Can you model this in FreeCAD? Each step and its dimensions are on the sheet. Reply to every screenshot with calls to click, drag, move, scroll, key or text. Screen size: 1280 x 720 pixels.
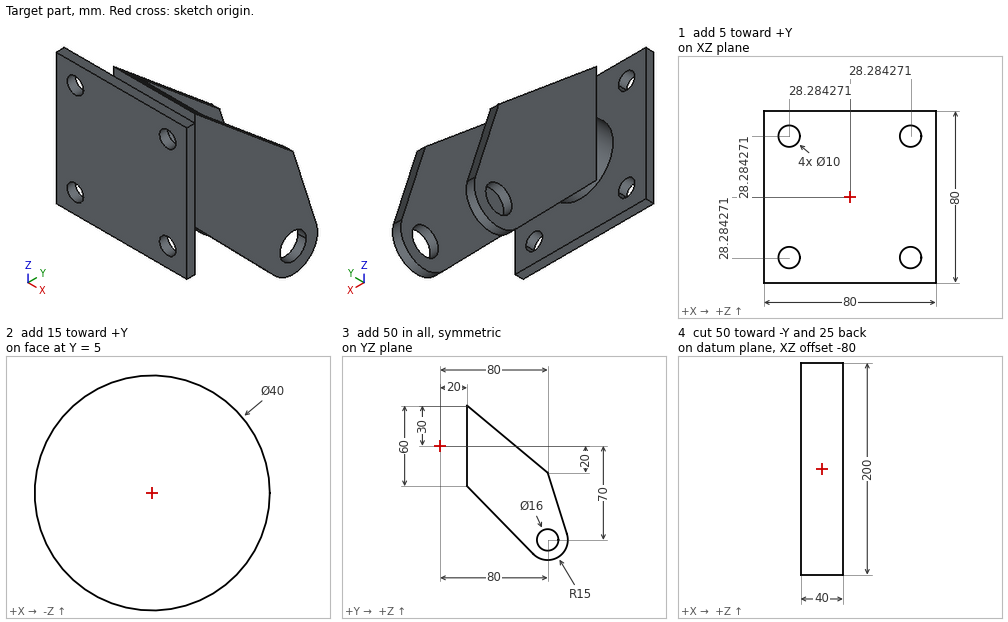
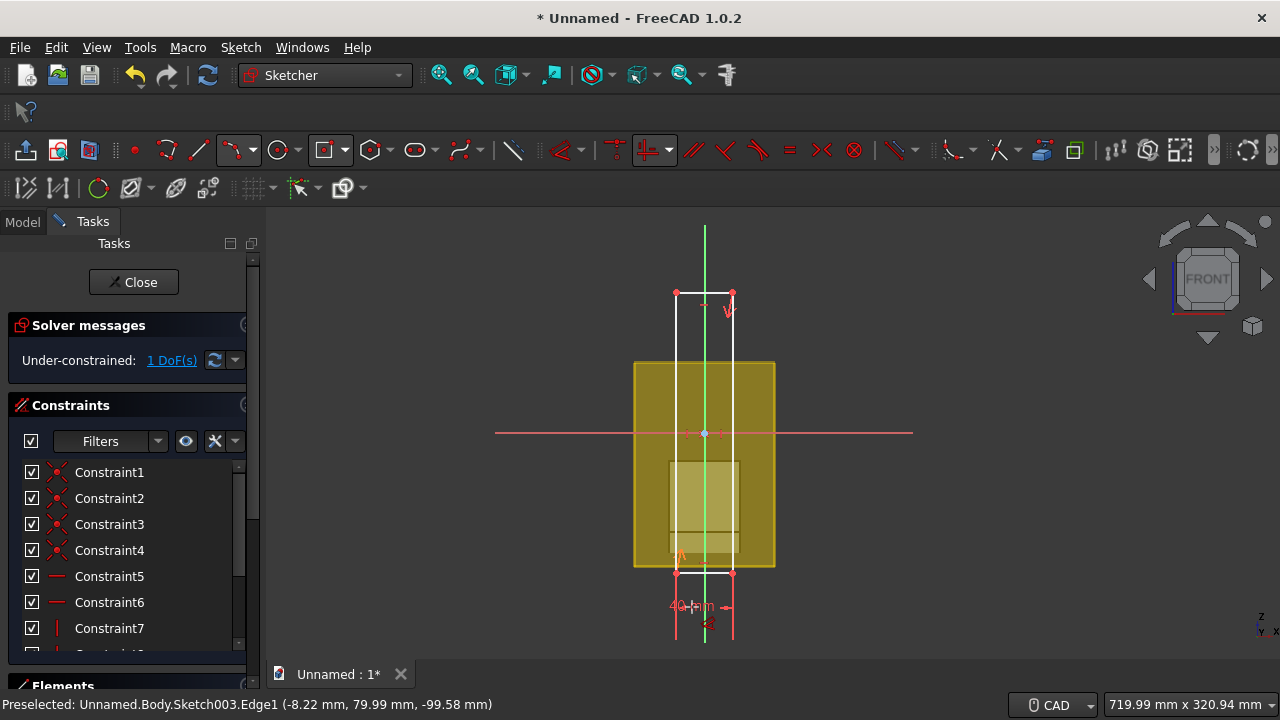
click(733, 489)
click(767, 369)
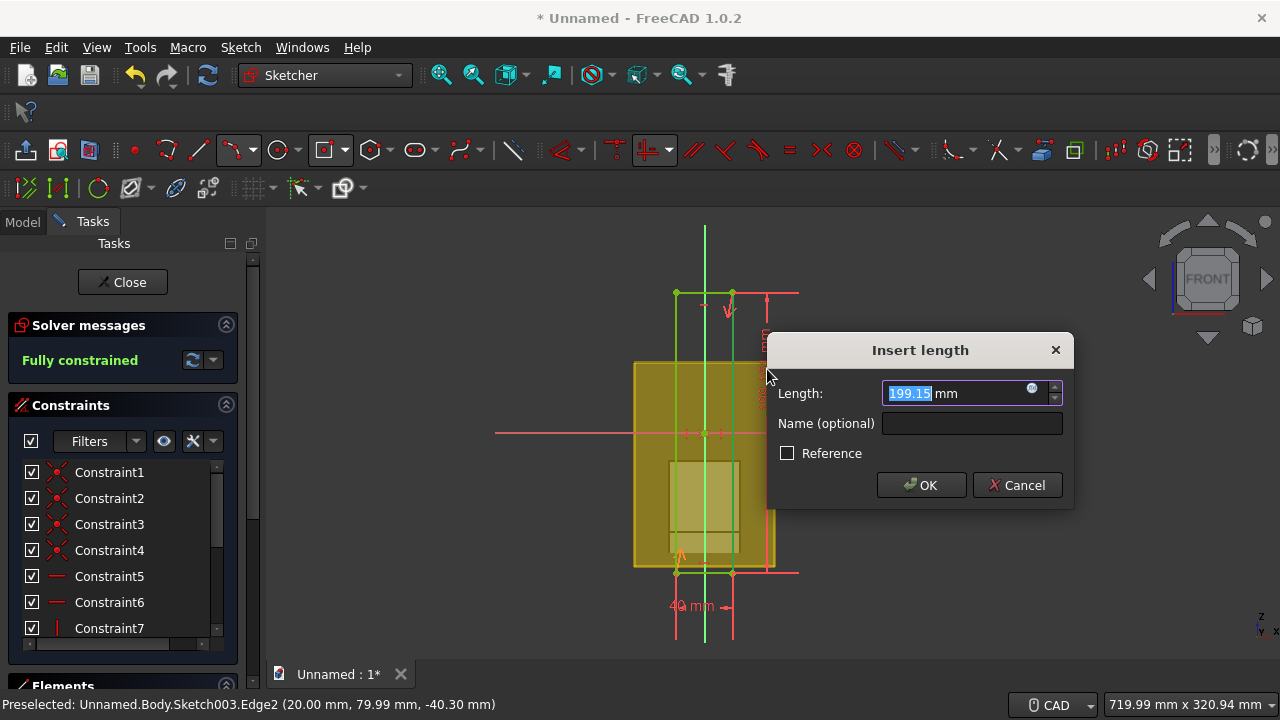
text(200)
key(Return)
key(Escape)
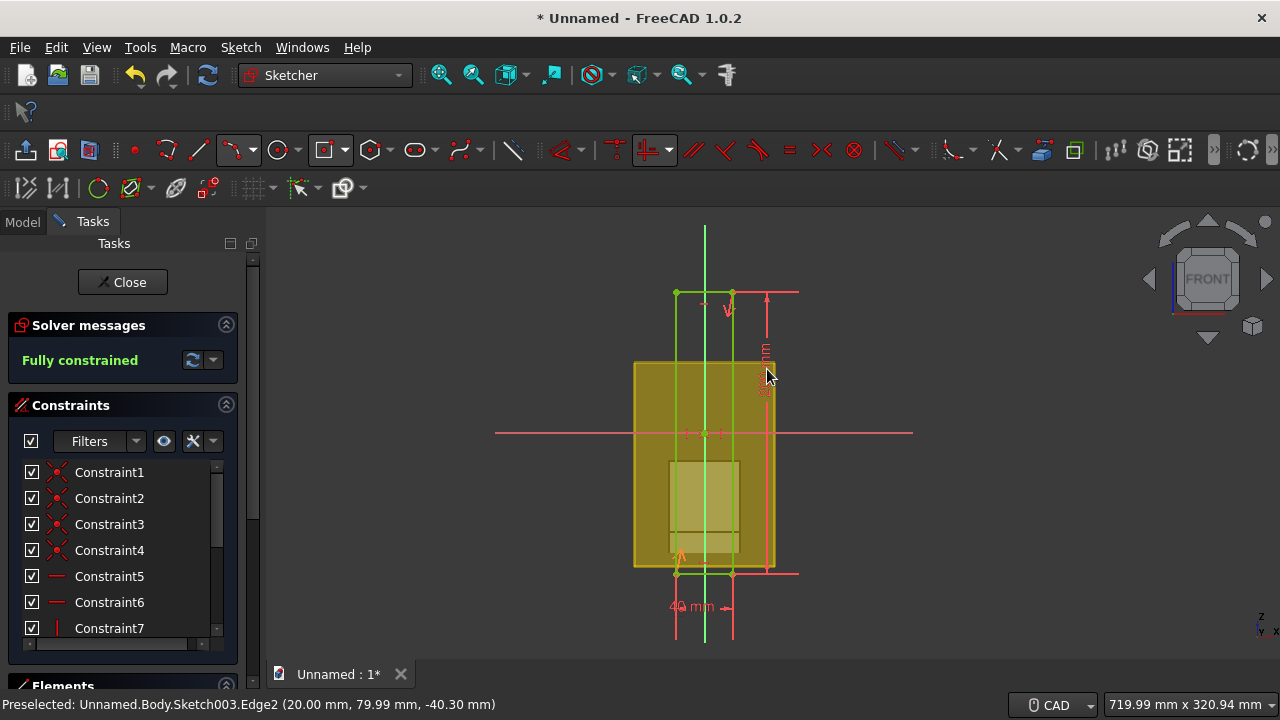
click(123, 282)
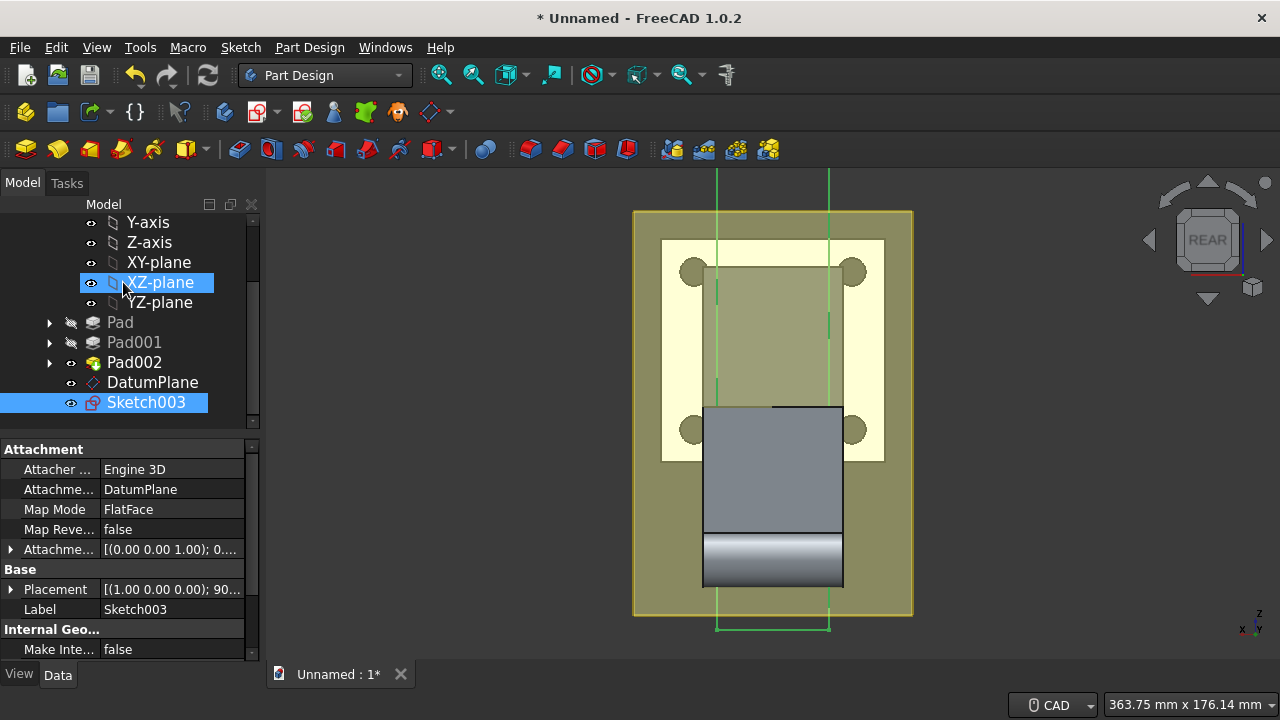
click(240, 150)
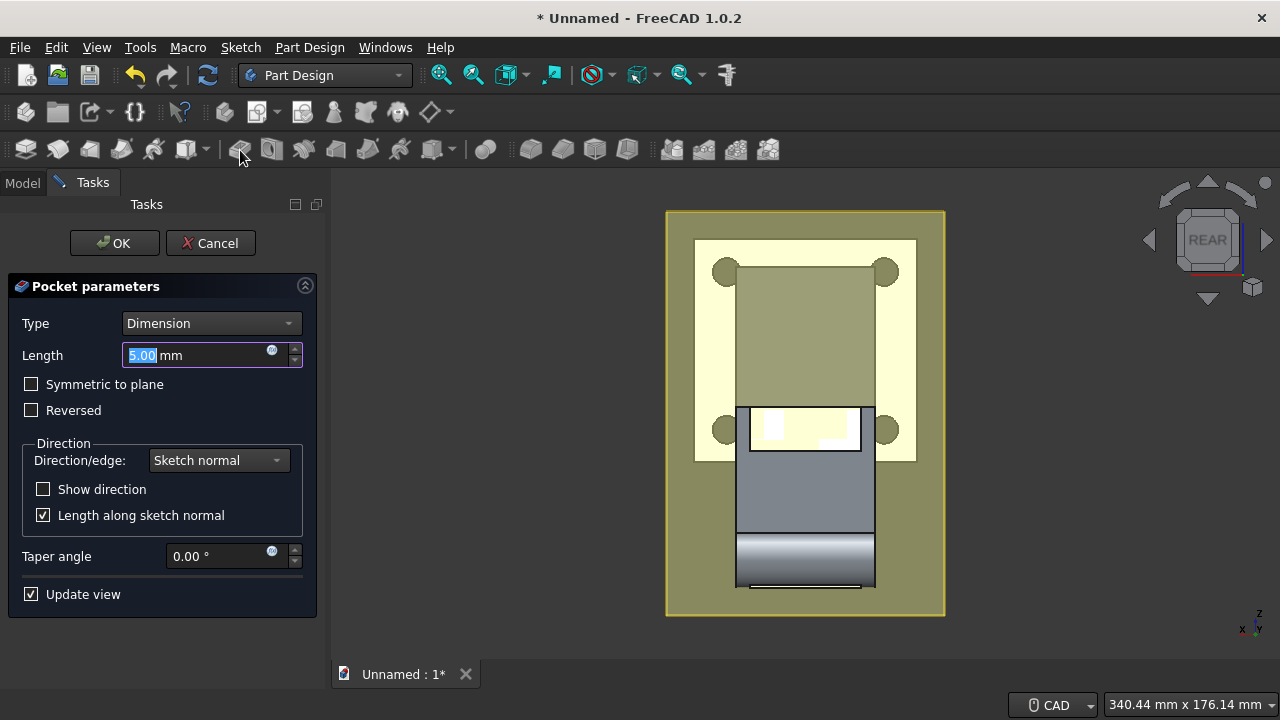
click(212, 324)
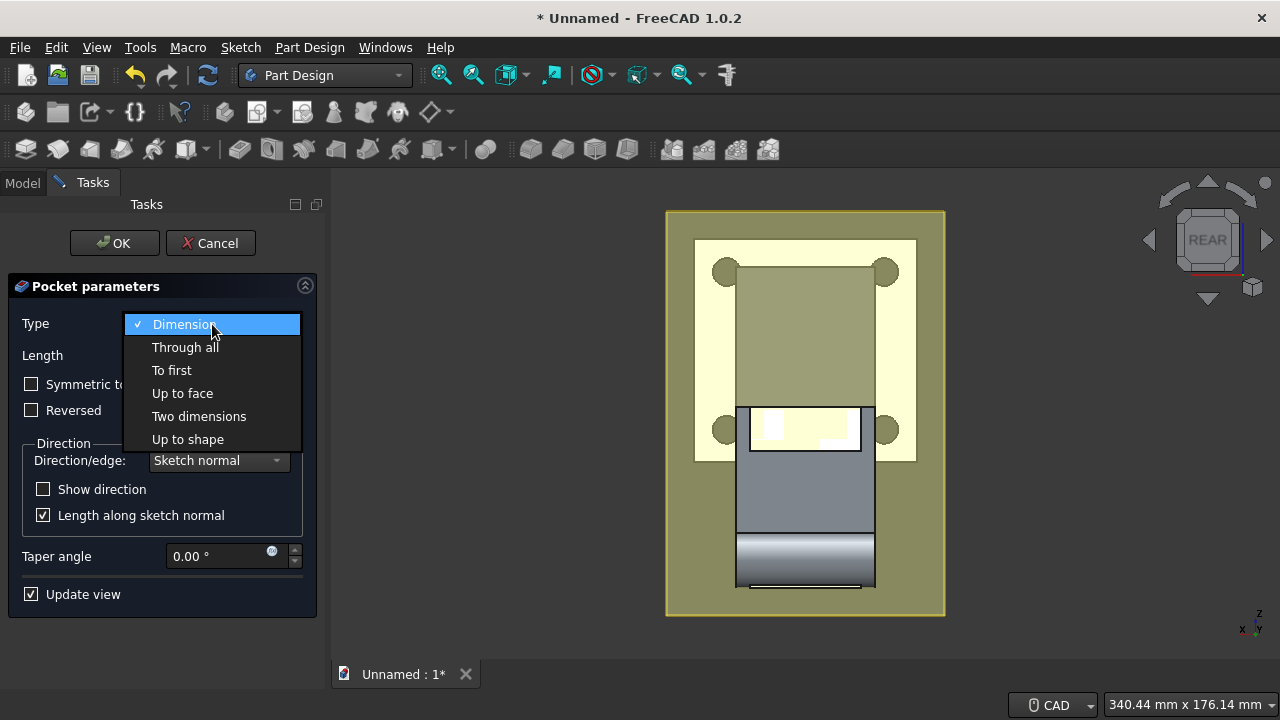
click(212, 416)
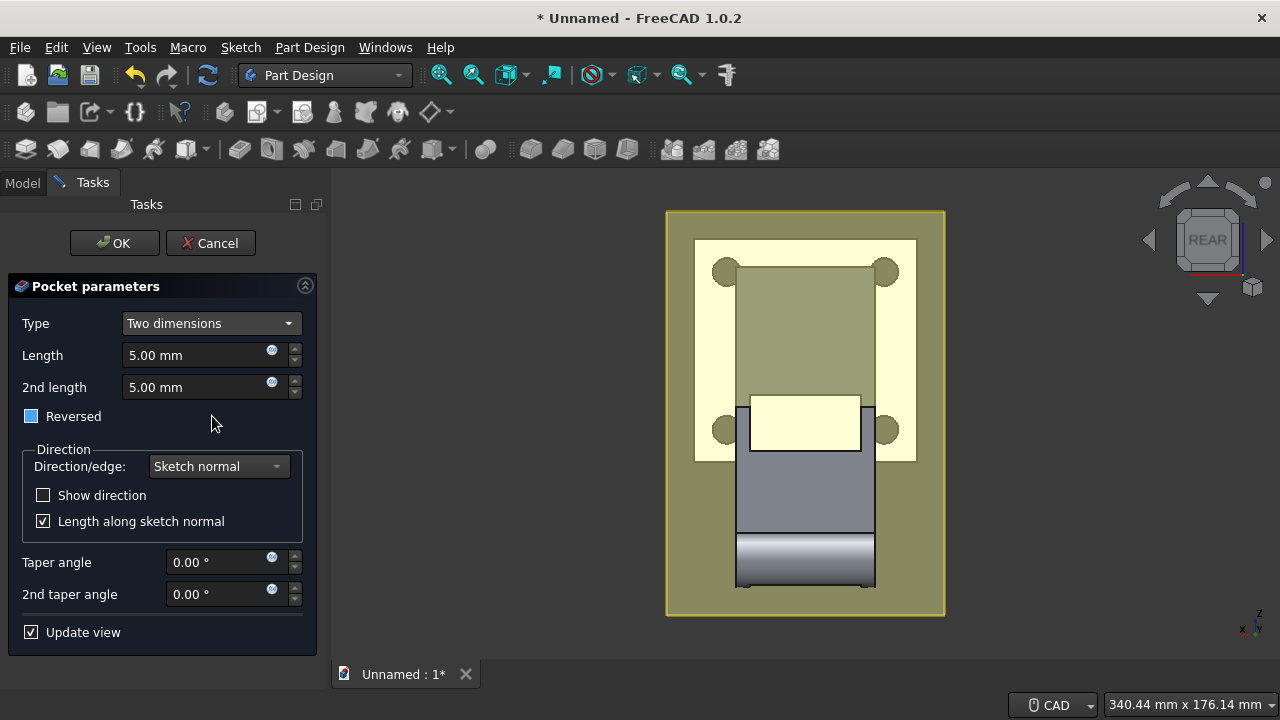
triple_click(204, 355)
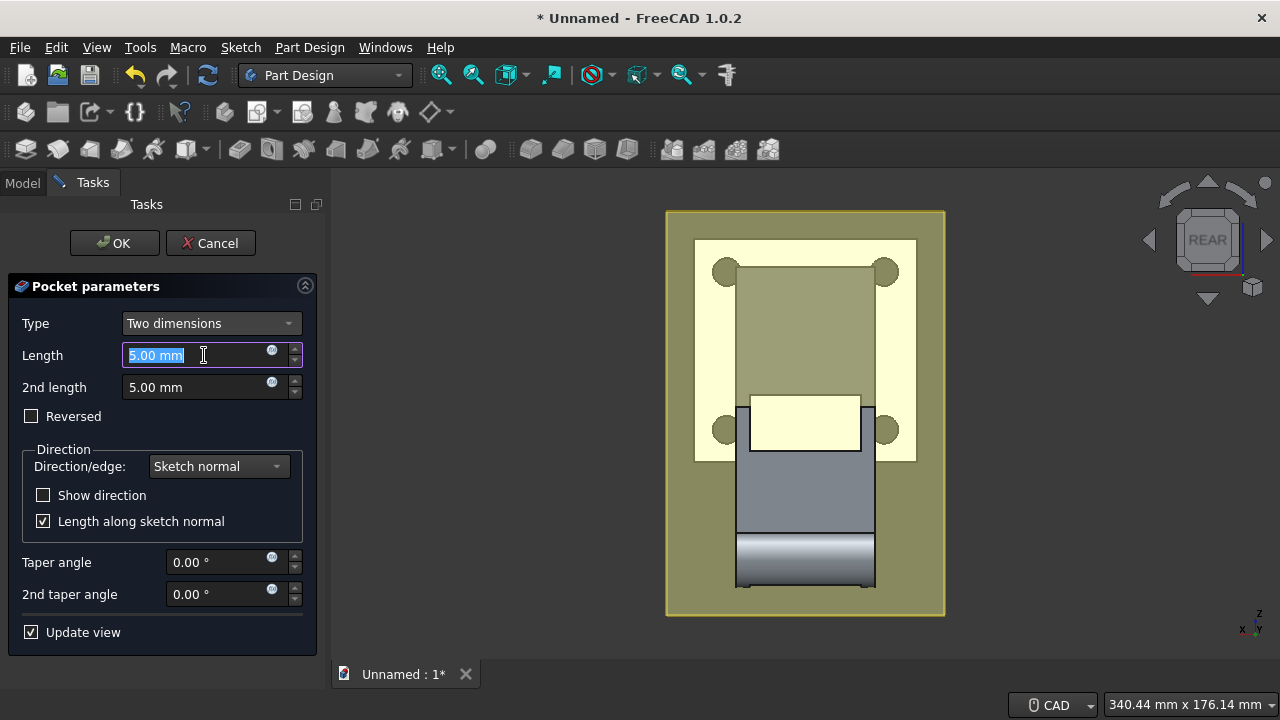
text(50)
key(Tab)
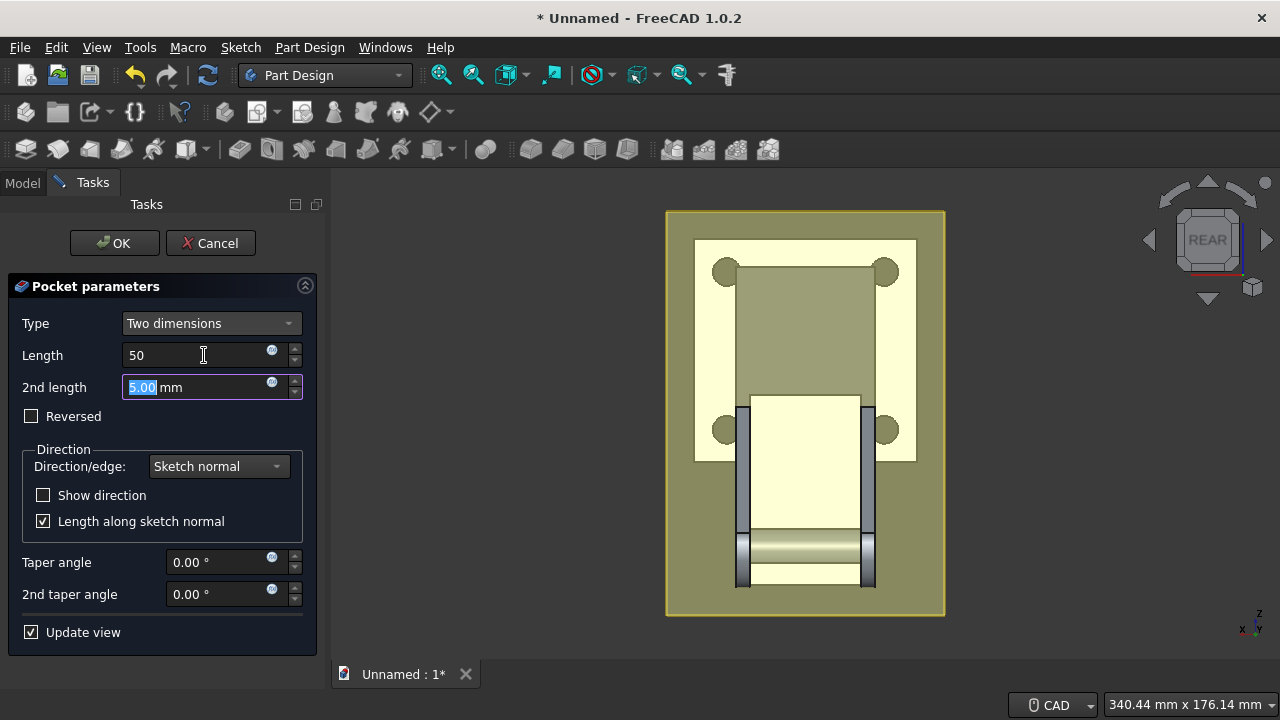
text(25)
key(Tab)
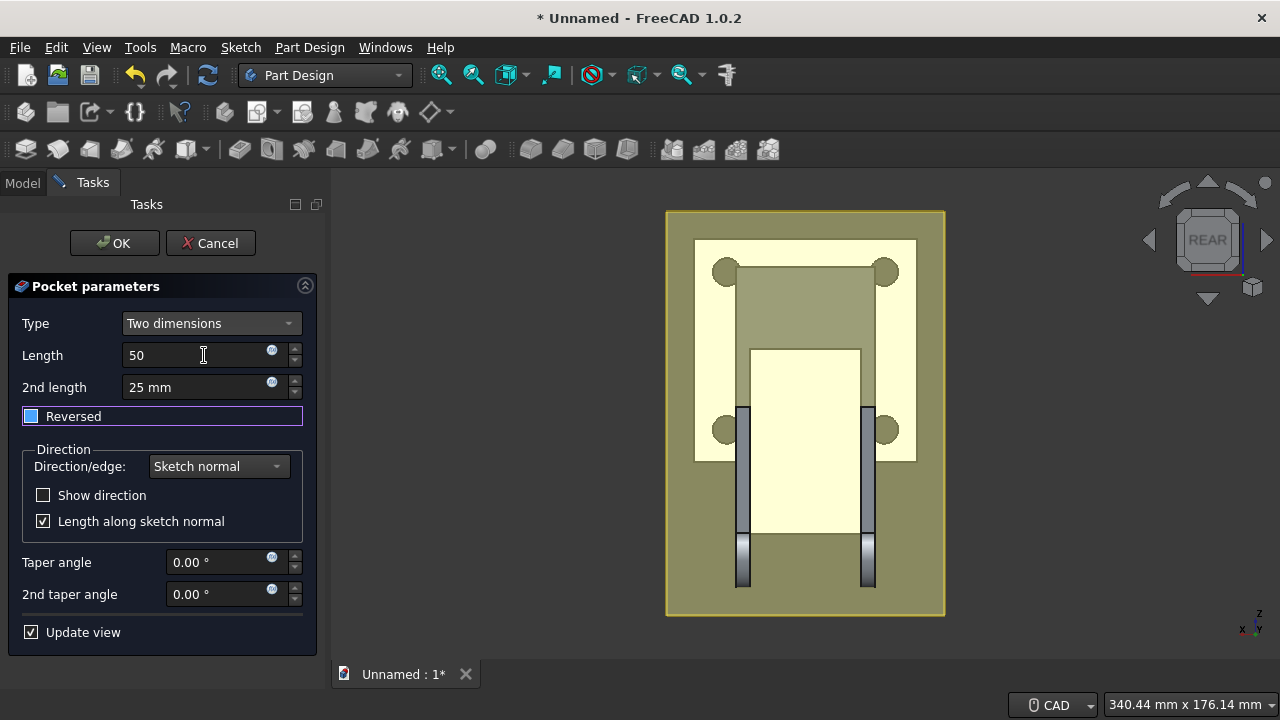
click(30, 416)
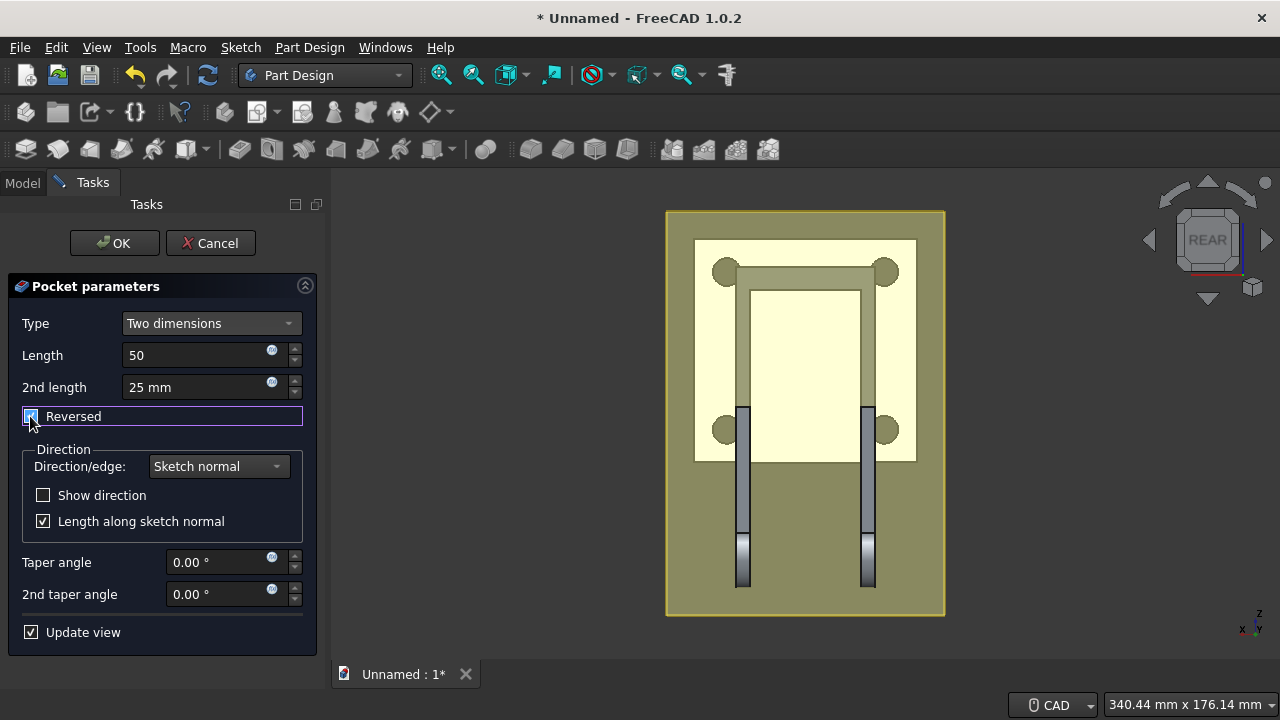
click(115, 243)